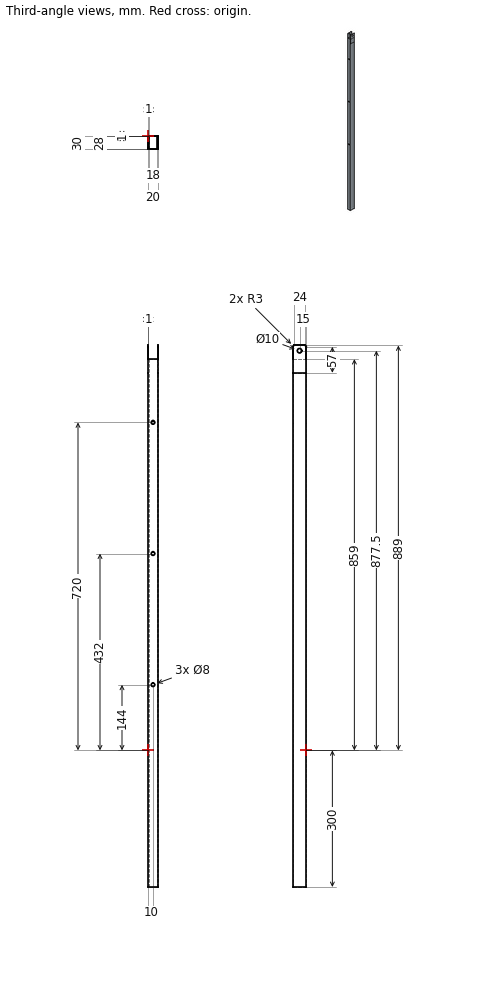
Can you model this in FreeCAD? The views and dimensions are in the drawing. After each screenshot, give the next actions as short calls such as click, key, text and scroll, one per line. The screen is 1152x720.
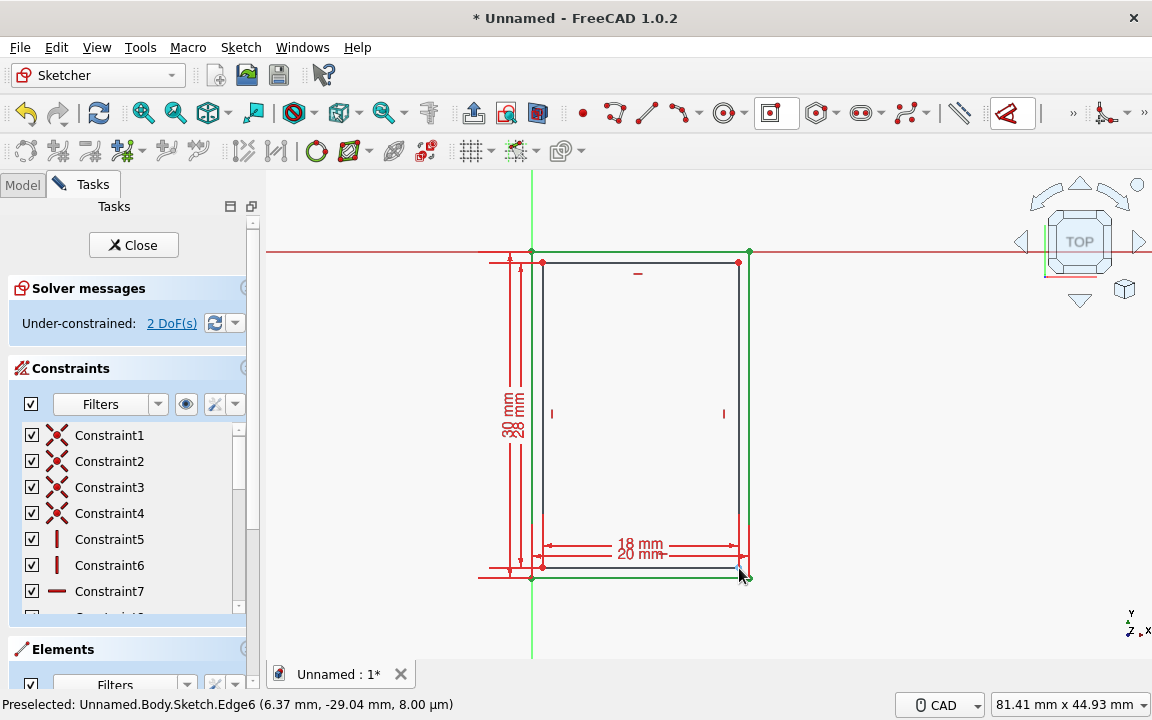
scroll(543, 263, up, 7)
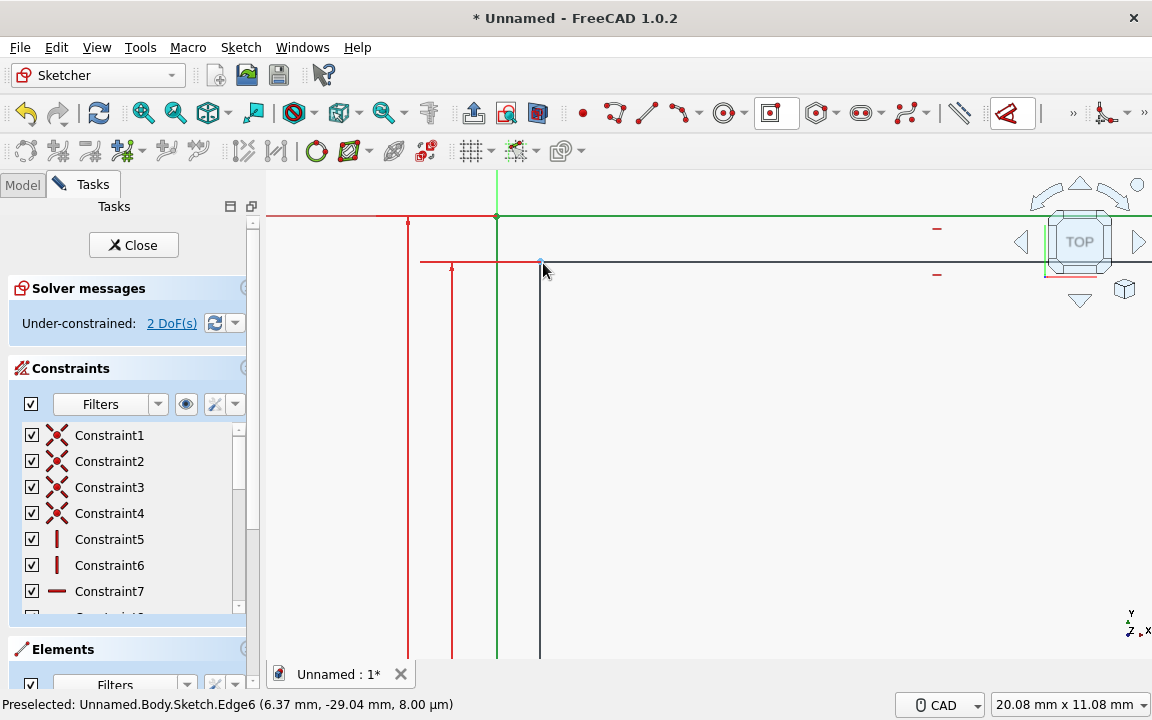
click(540, 262)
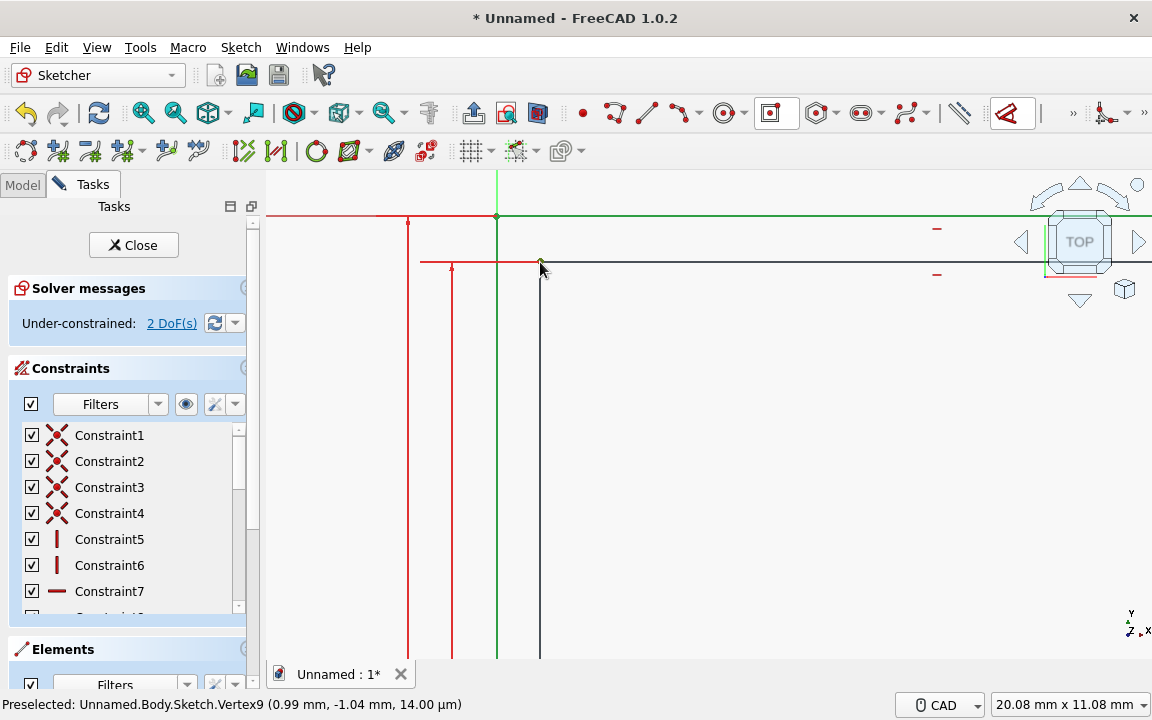
key(l)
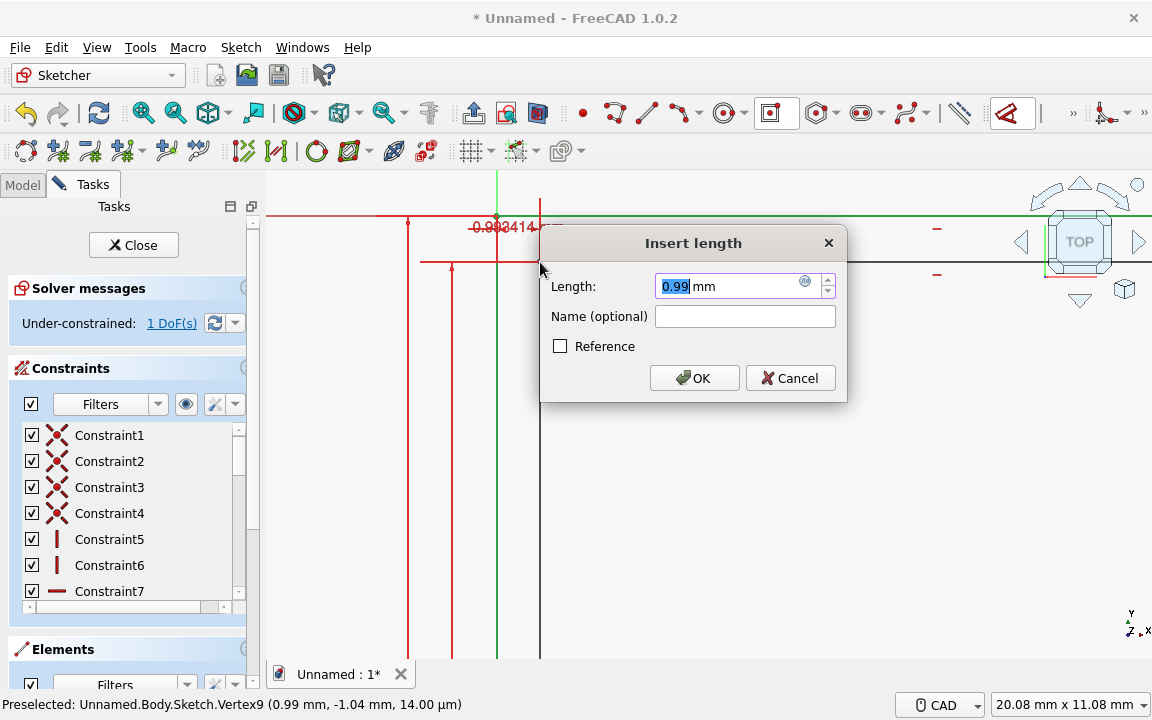
text(1)
key(Return)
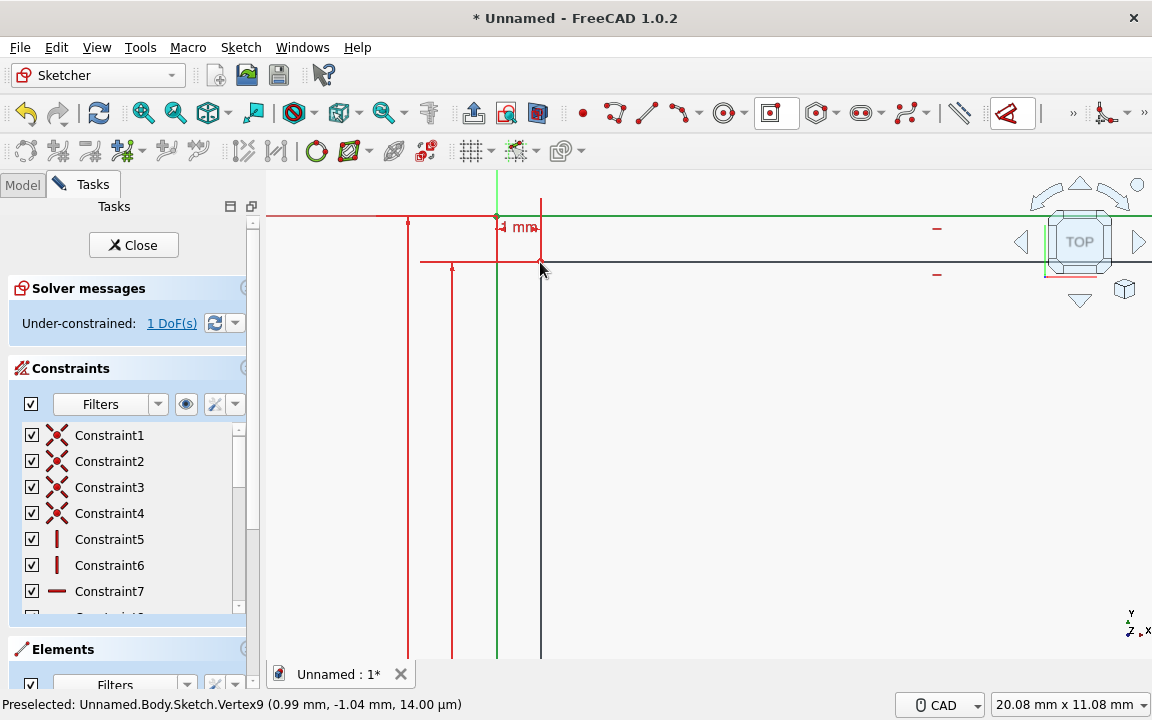
click(541, 262)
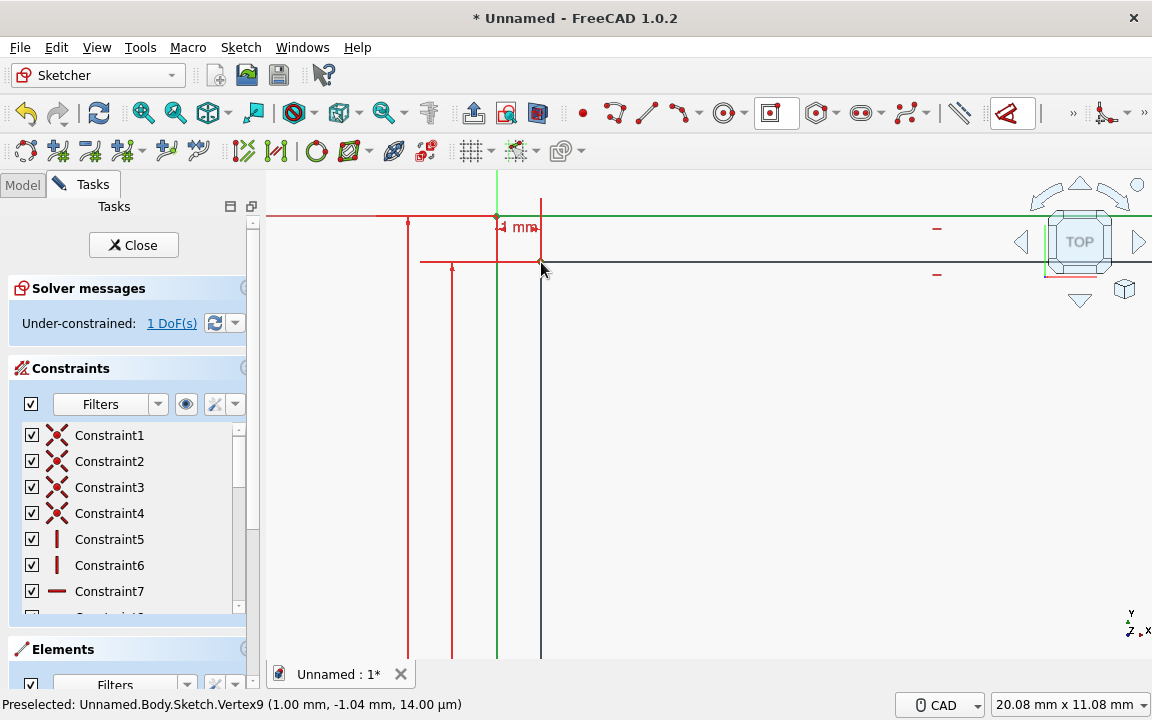
key(i)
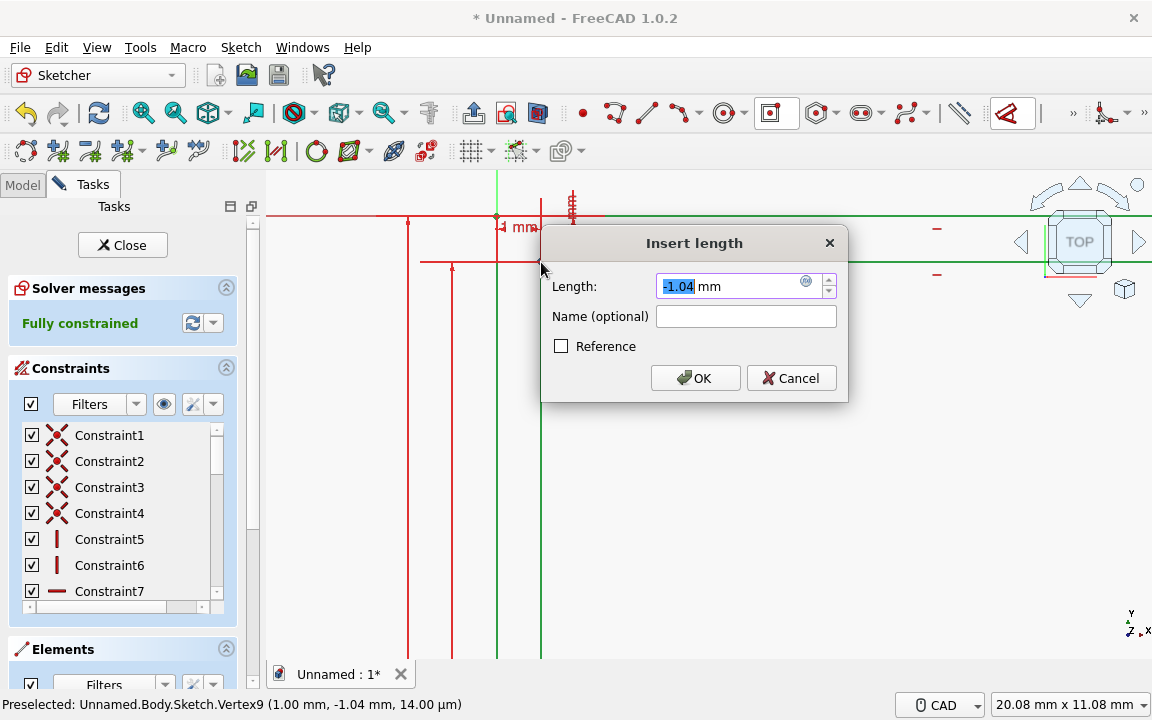
text(-1)
key(Return)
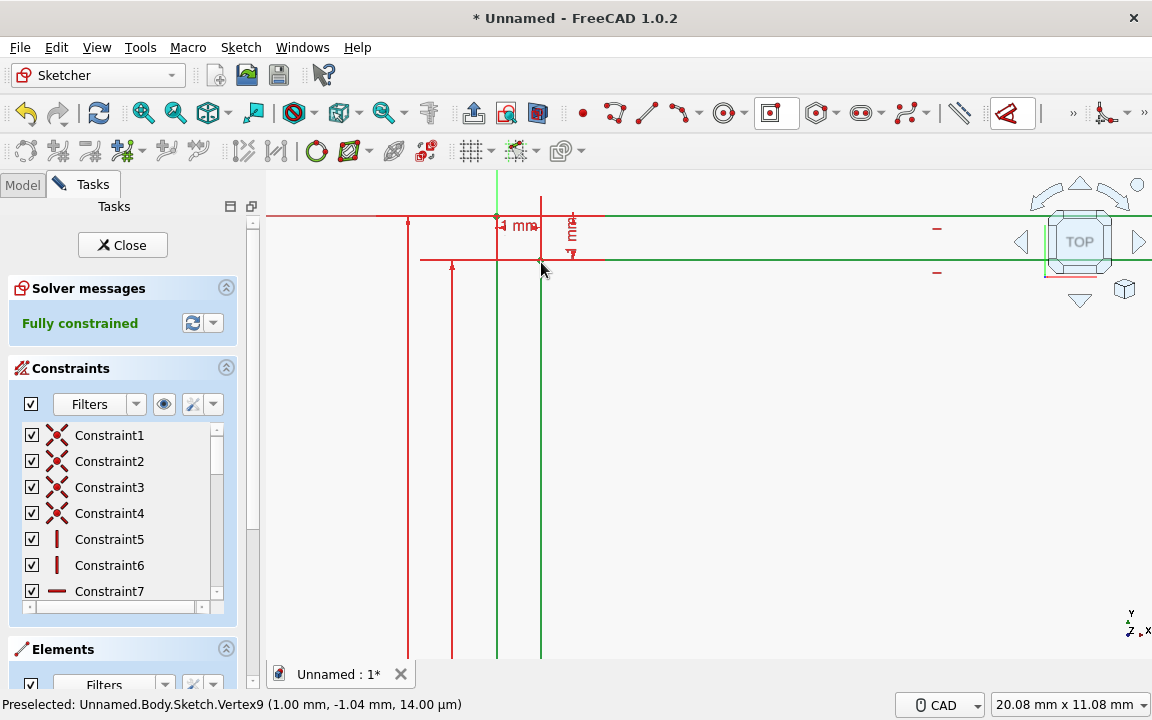
click(123, 245)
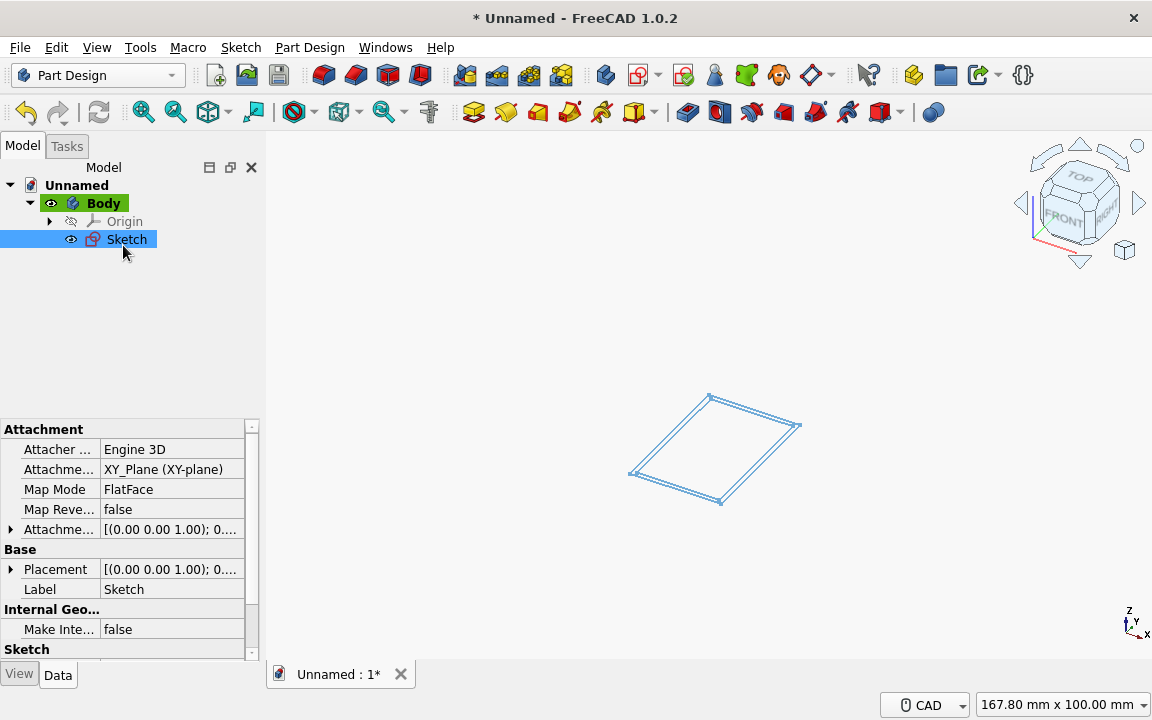
click(474, 112)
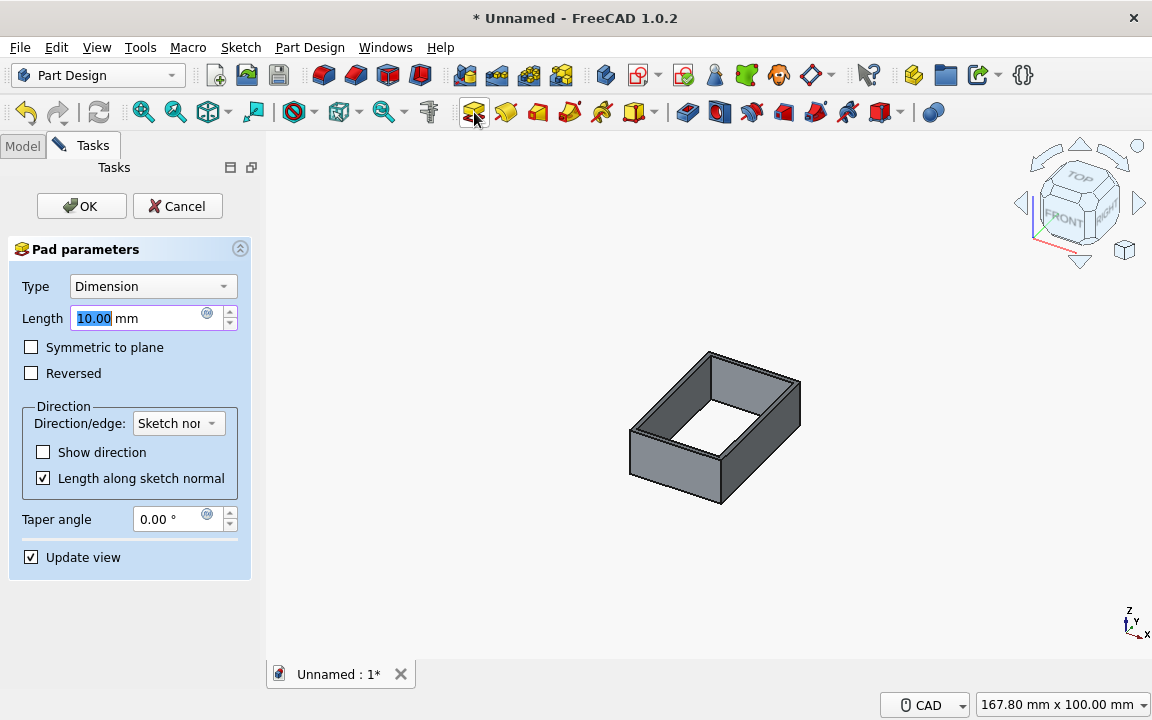
text(859)
key(Tab)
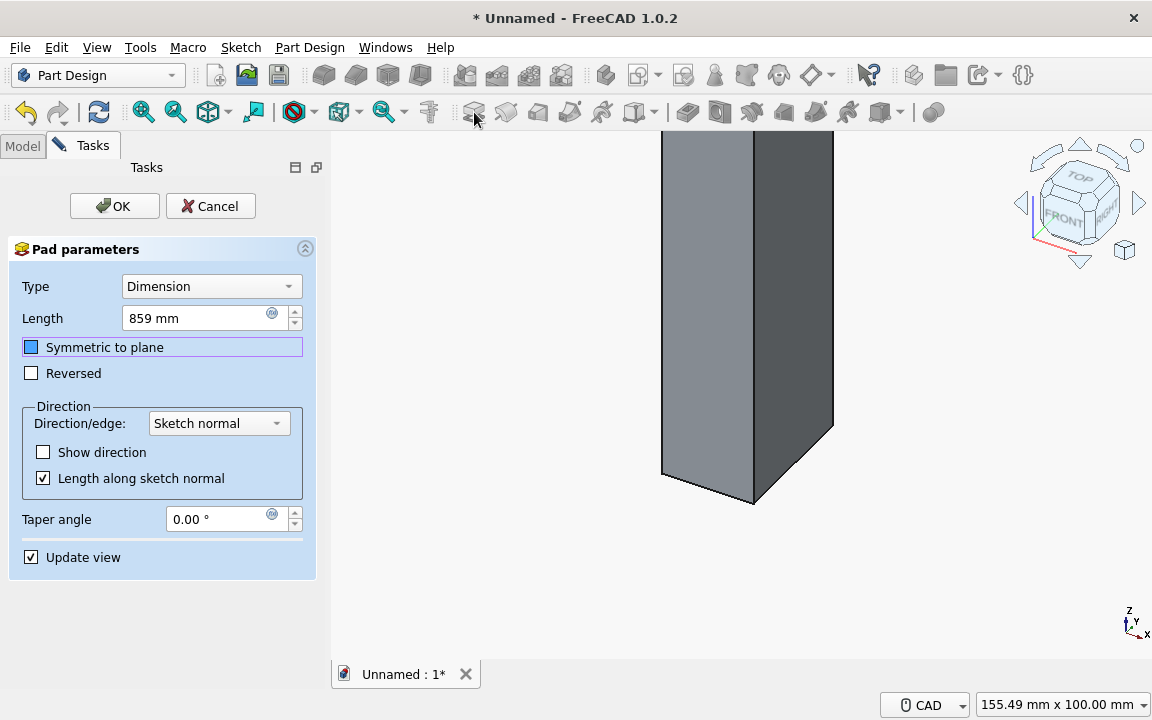
click(115, 206)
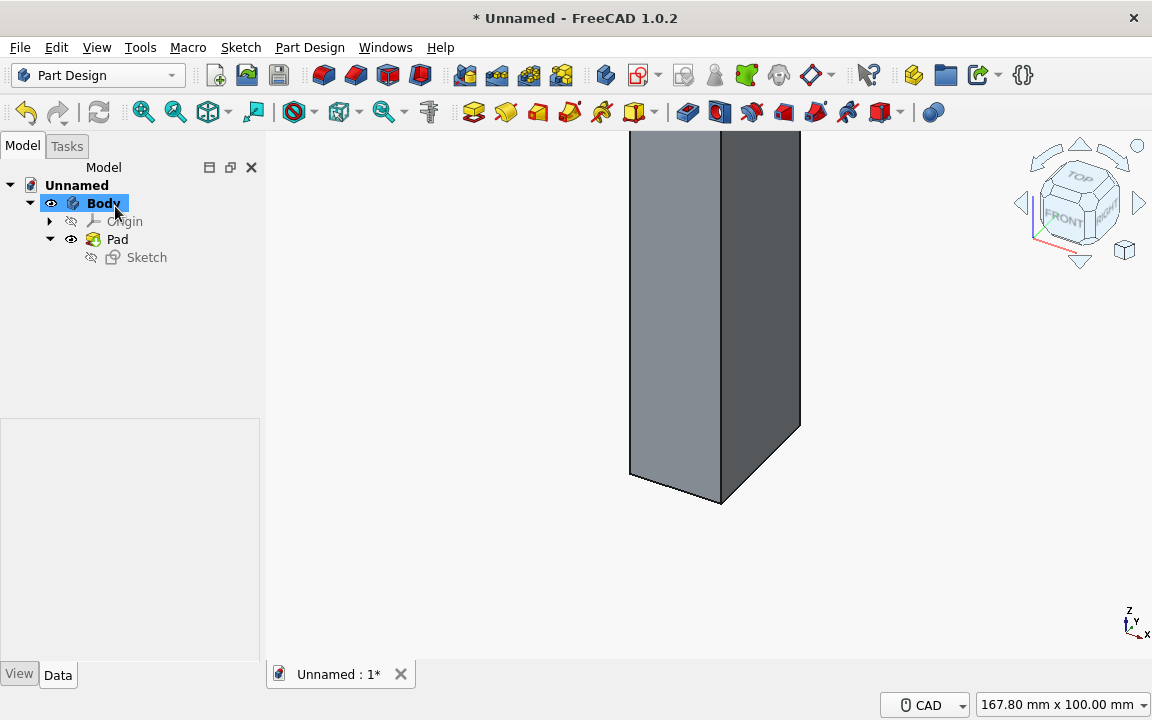
key(v)
key(f)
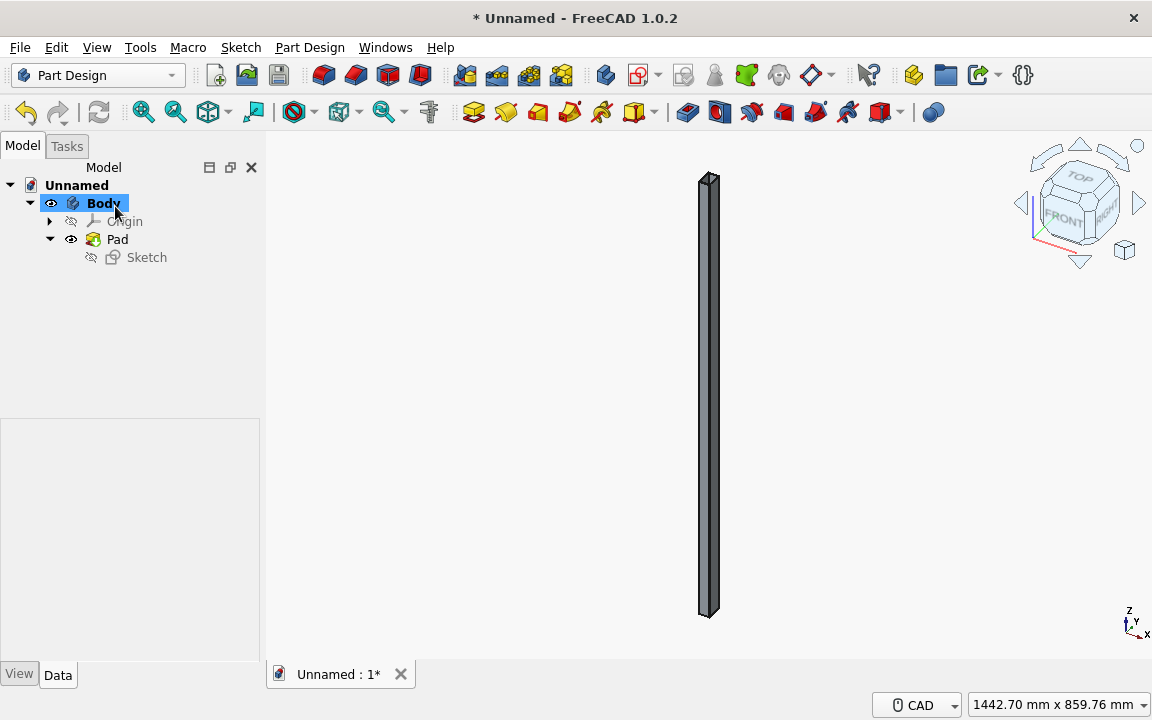
key(6)